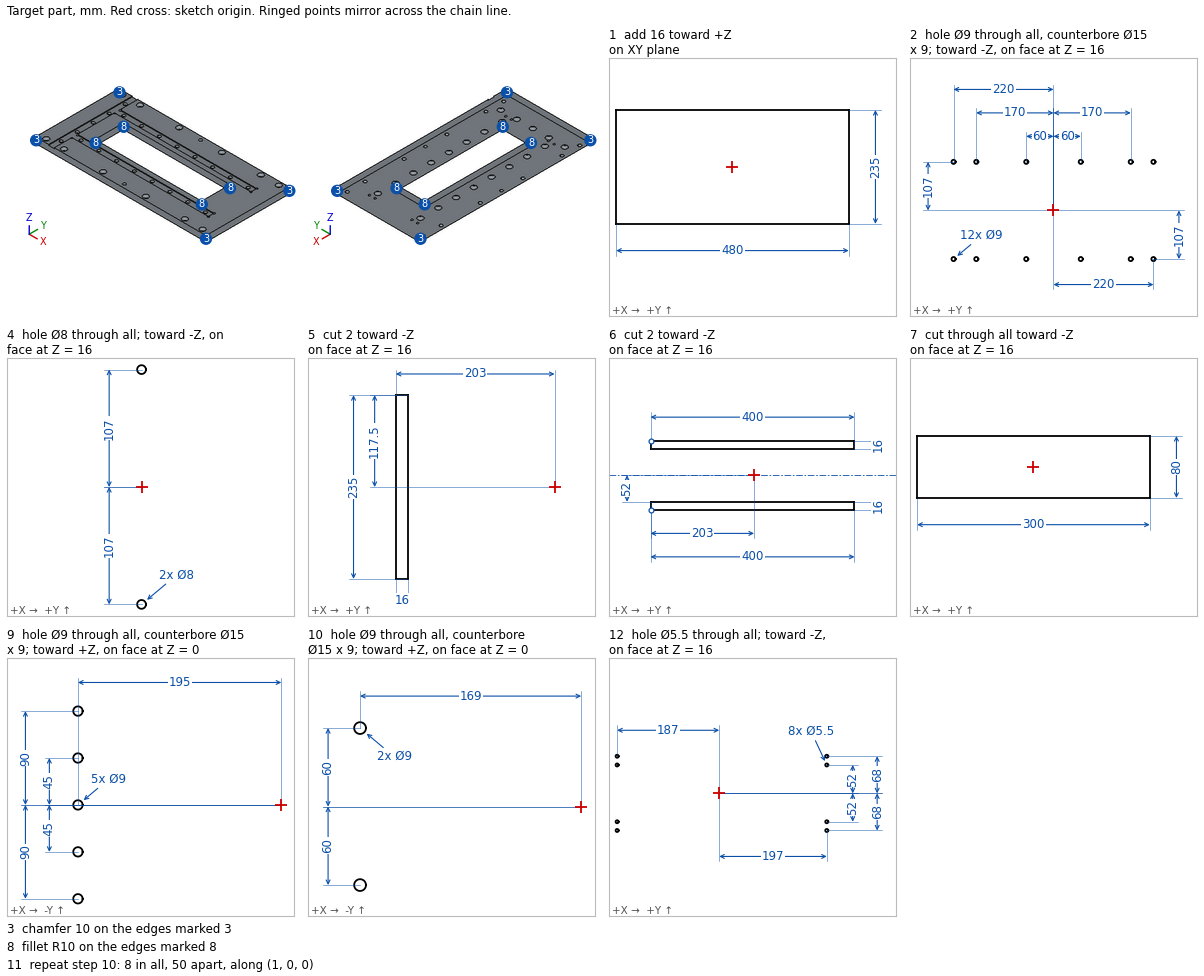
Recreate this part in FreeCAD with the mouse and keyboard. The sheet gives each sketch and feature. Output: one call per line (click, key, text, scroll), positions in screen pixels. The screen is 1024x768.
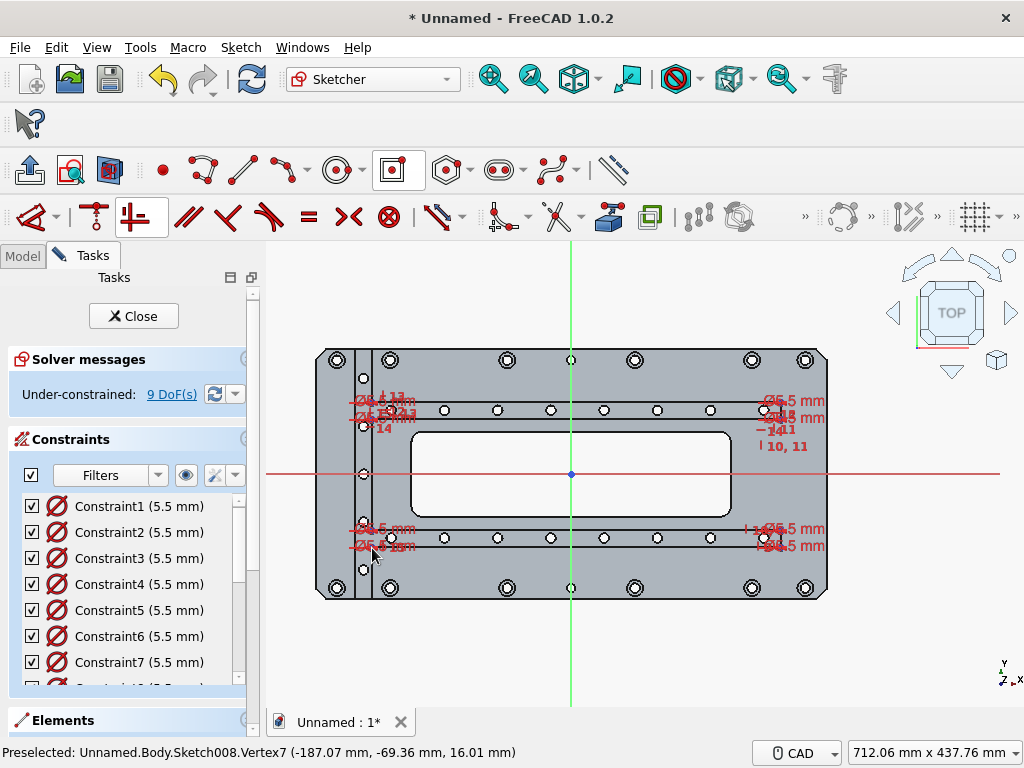
click(781, 548)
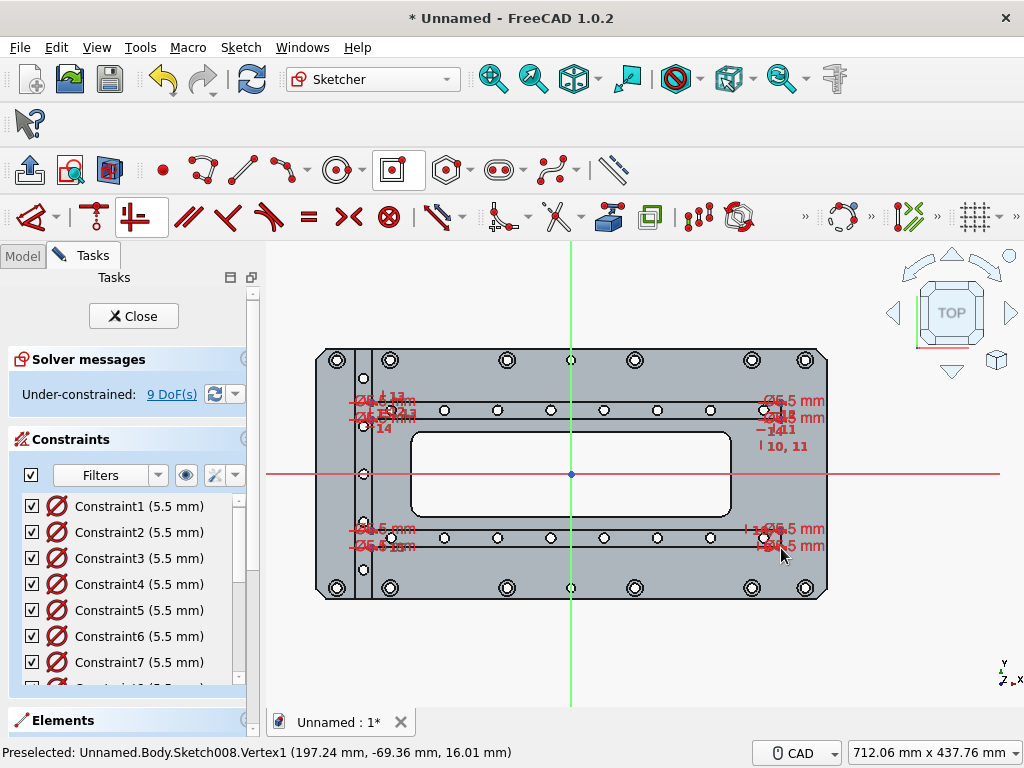
click(372, 548)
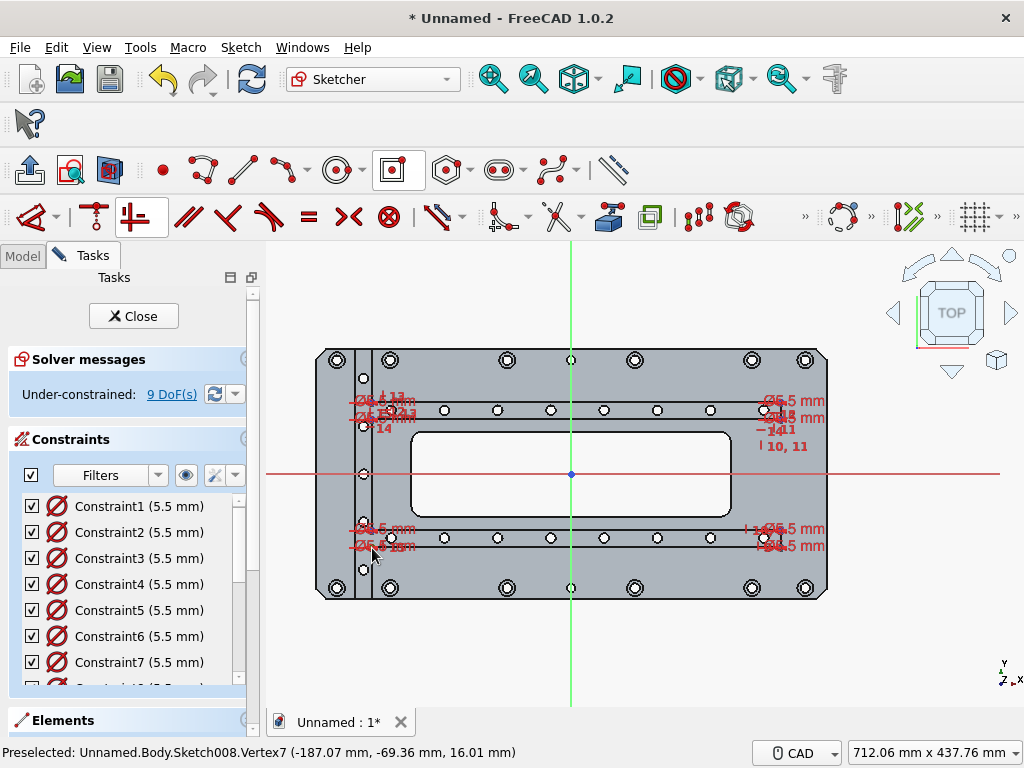
click(162, 218)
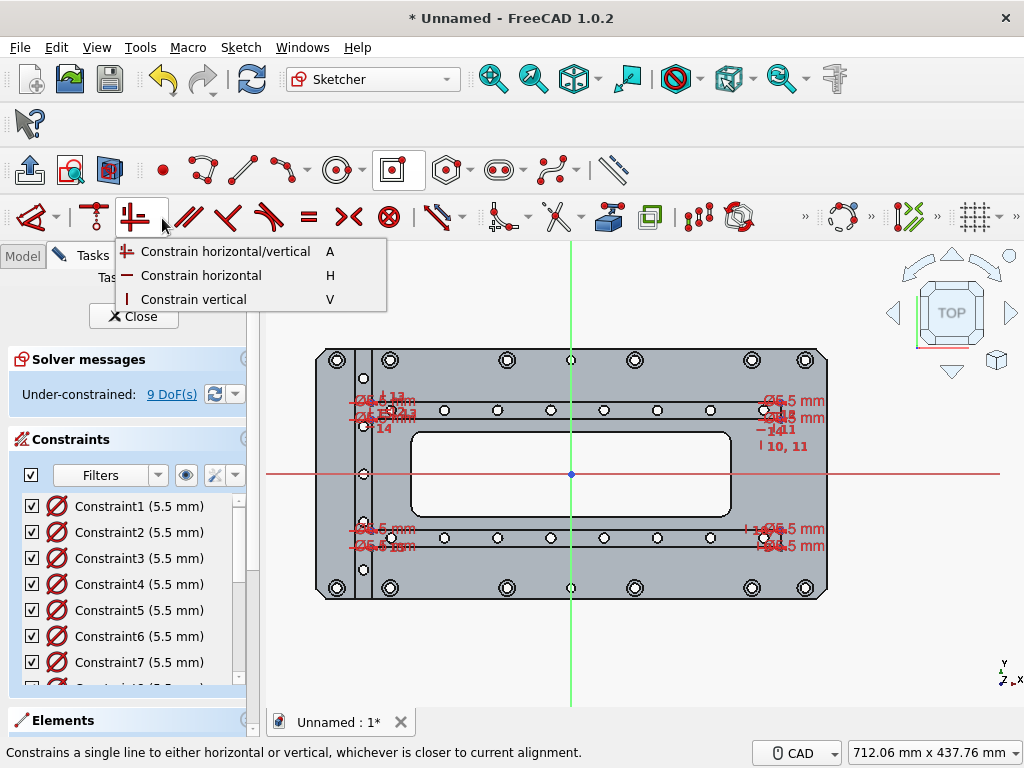
click(251, 275)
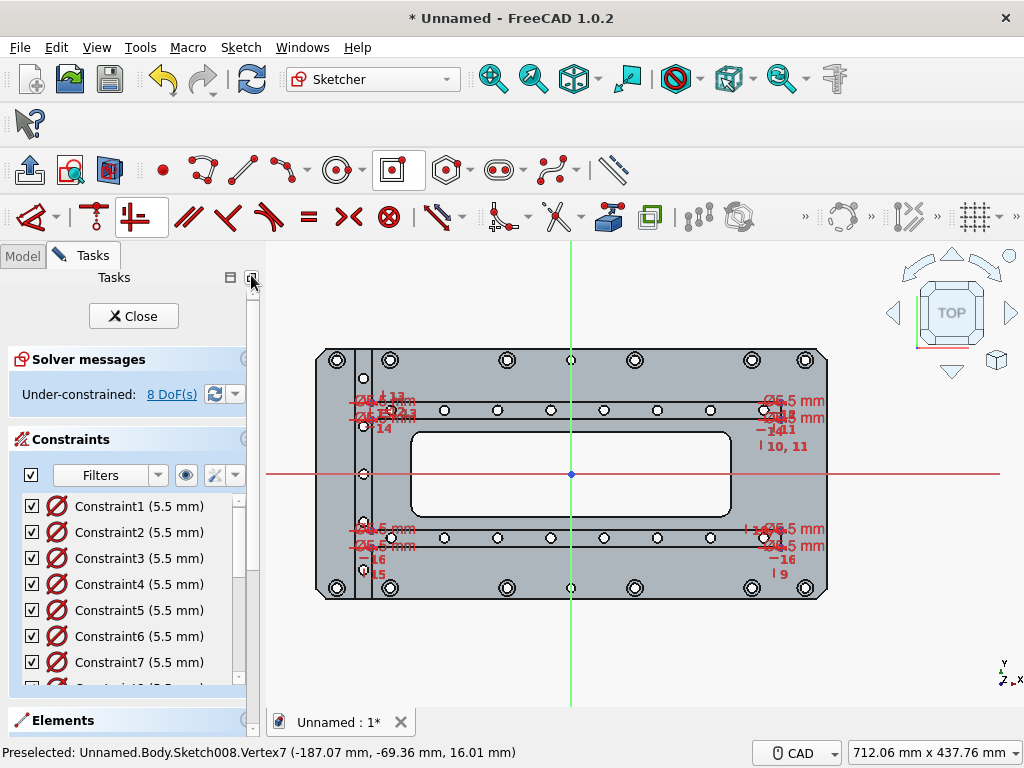
click(372, 548)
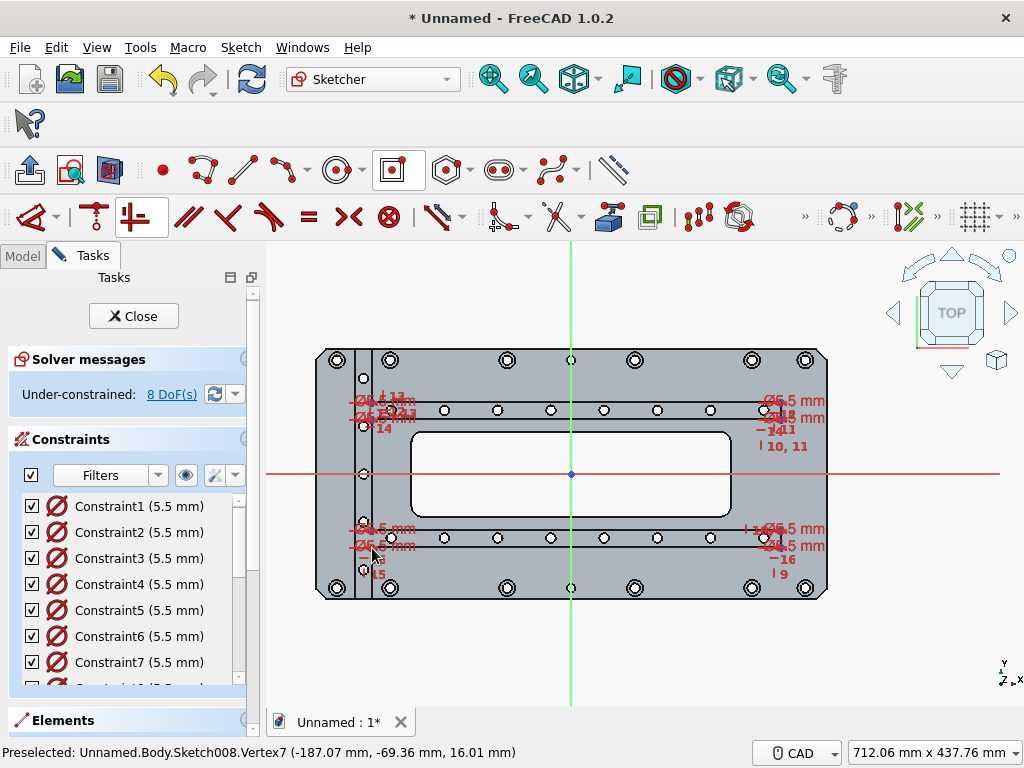
click(372, 531)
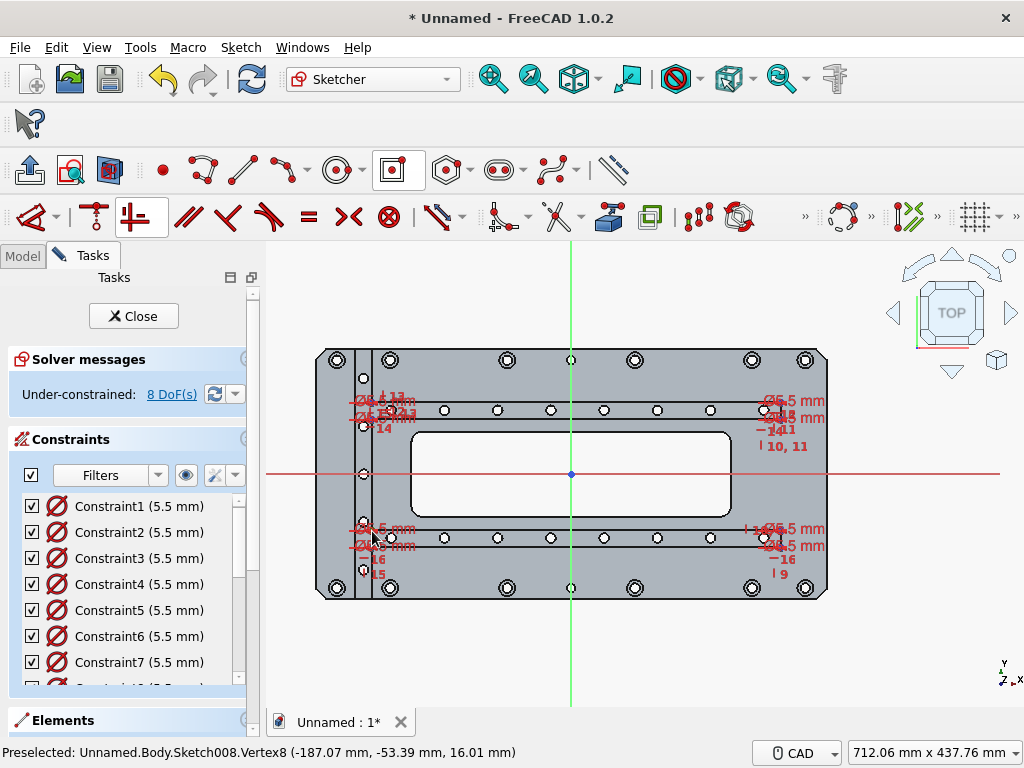
key(v)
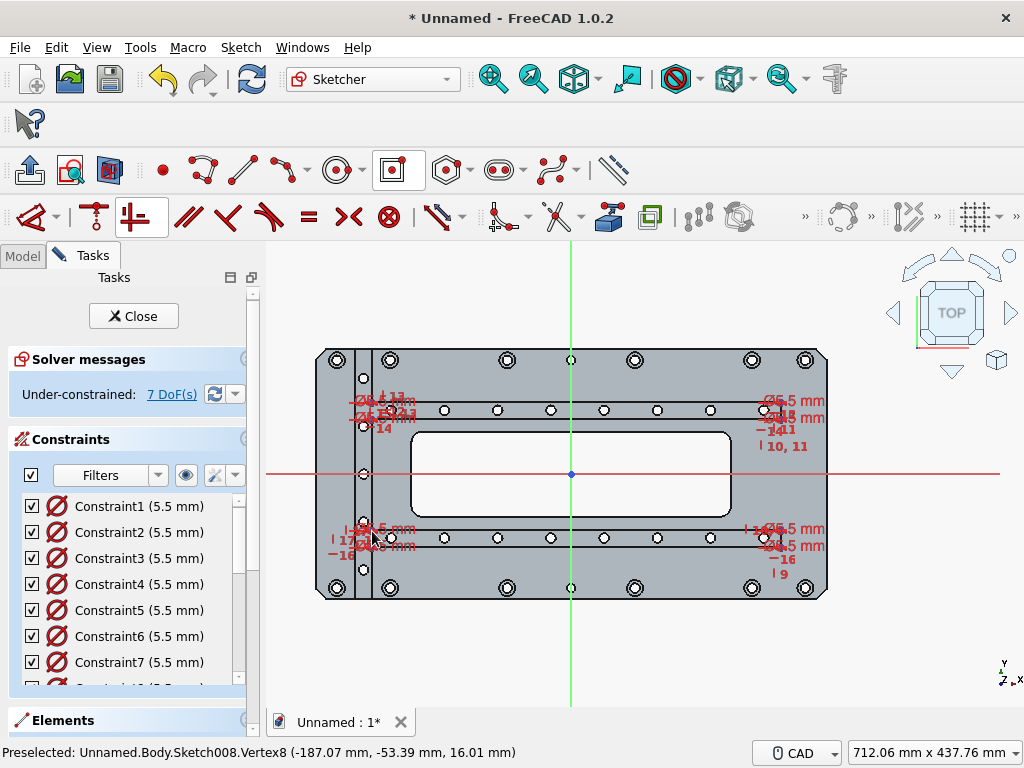
click(781, 531)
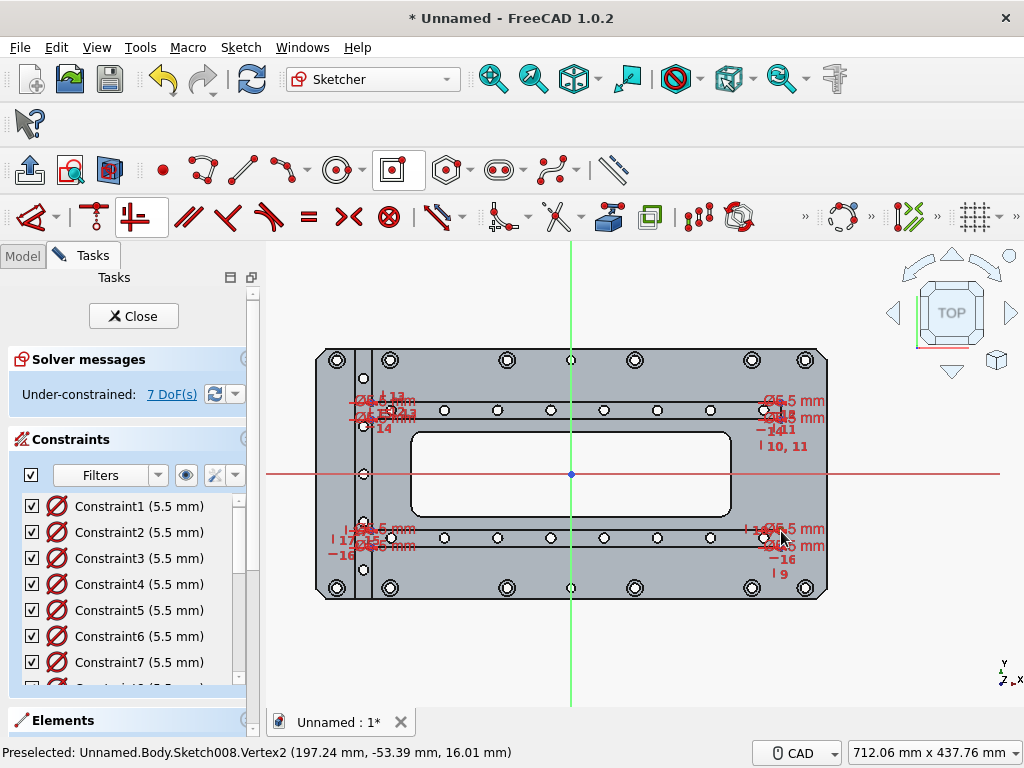
click(372, 531)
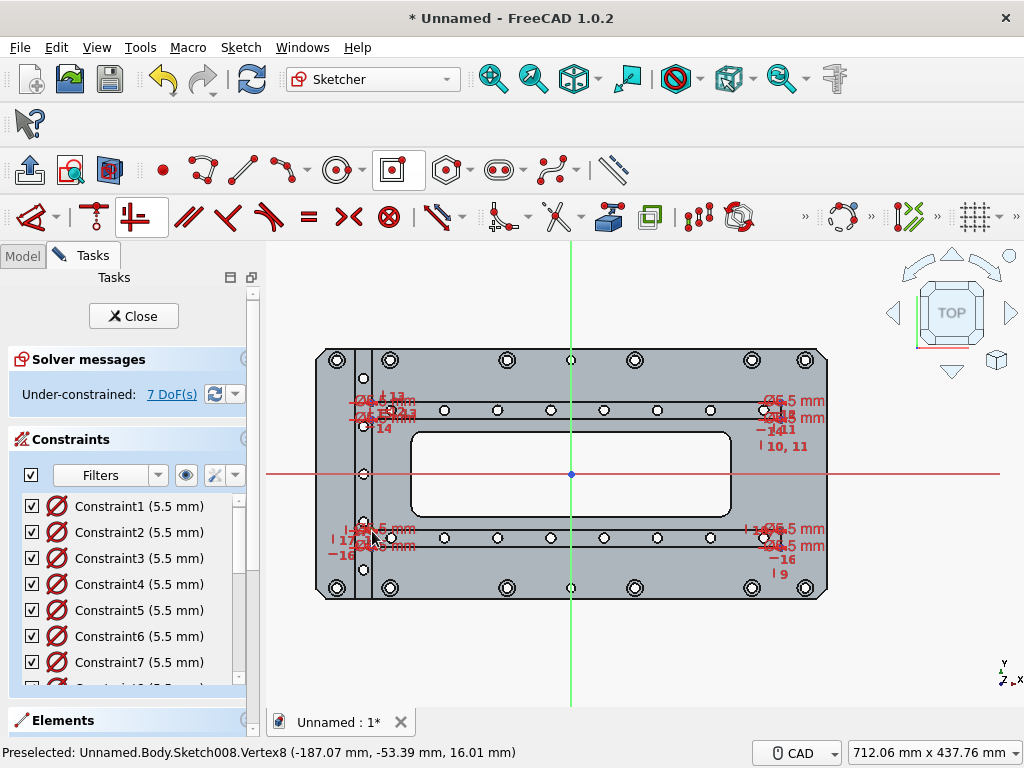
key(h)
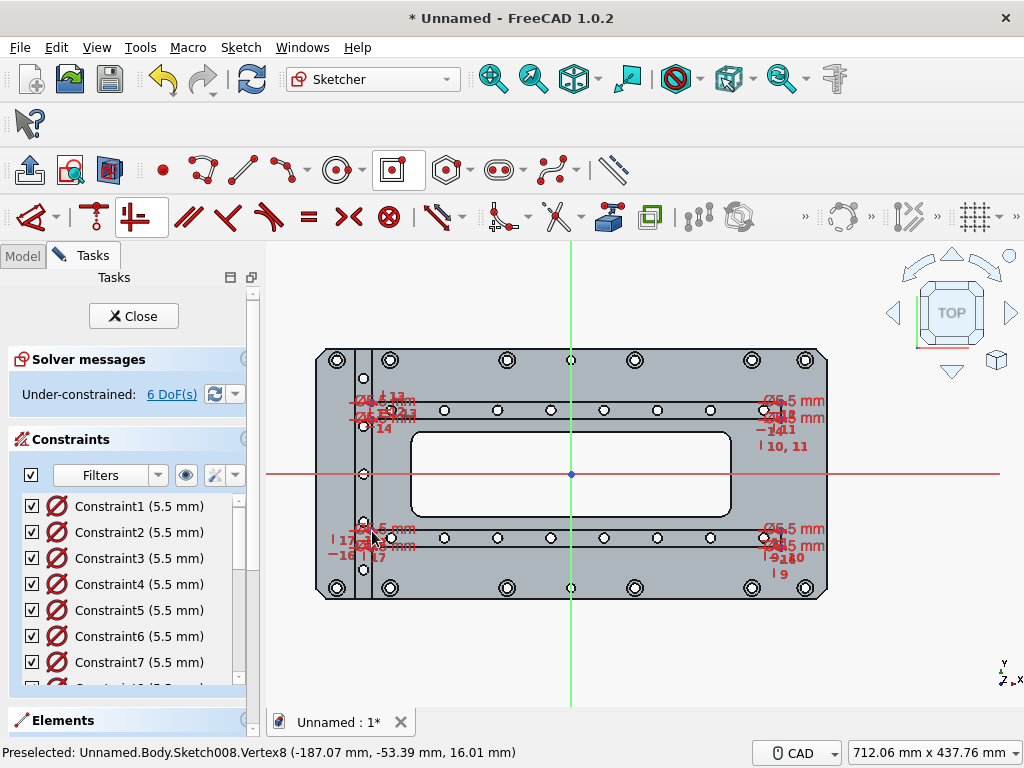
click(32, 218)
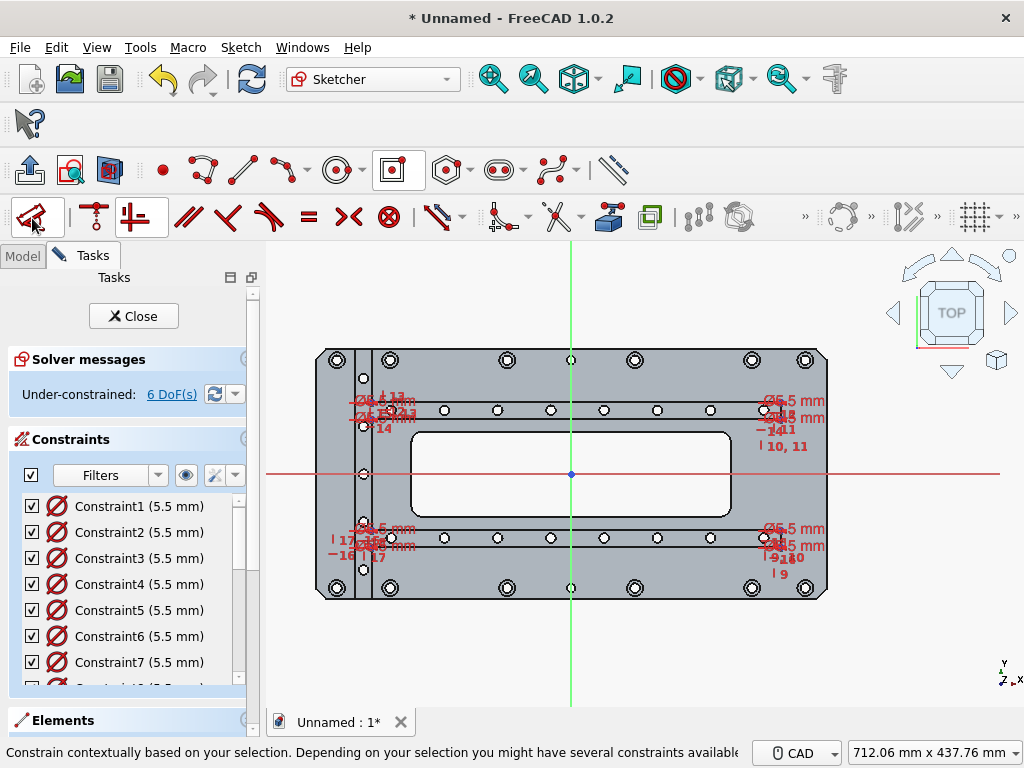
click(781, 548)
click(815, 511)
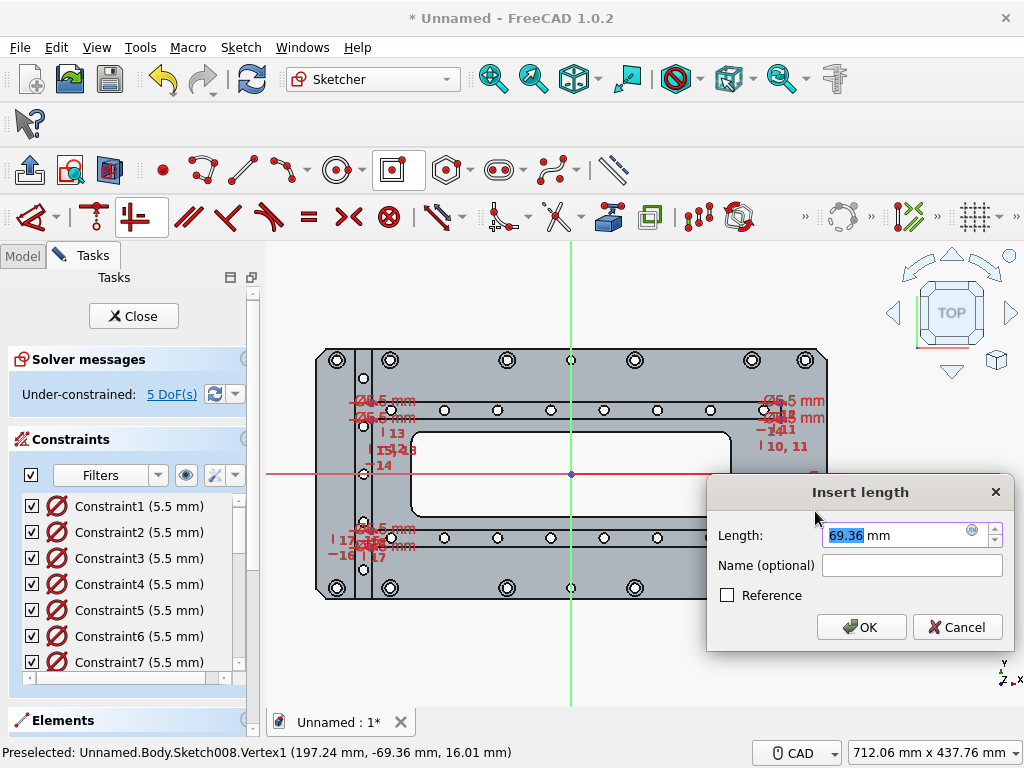
text(68)
key(Return)